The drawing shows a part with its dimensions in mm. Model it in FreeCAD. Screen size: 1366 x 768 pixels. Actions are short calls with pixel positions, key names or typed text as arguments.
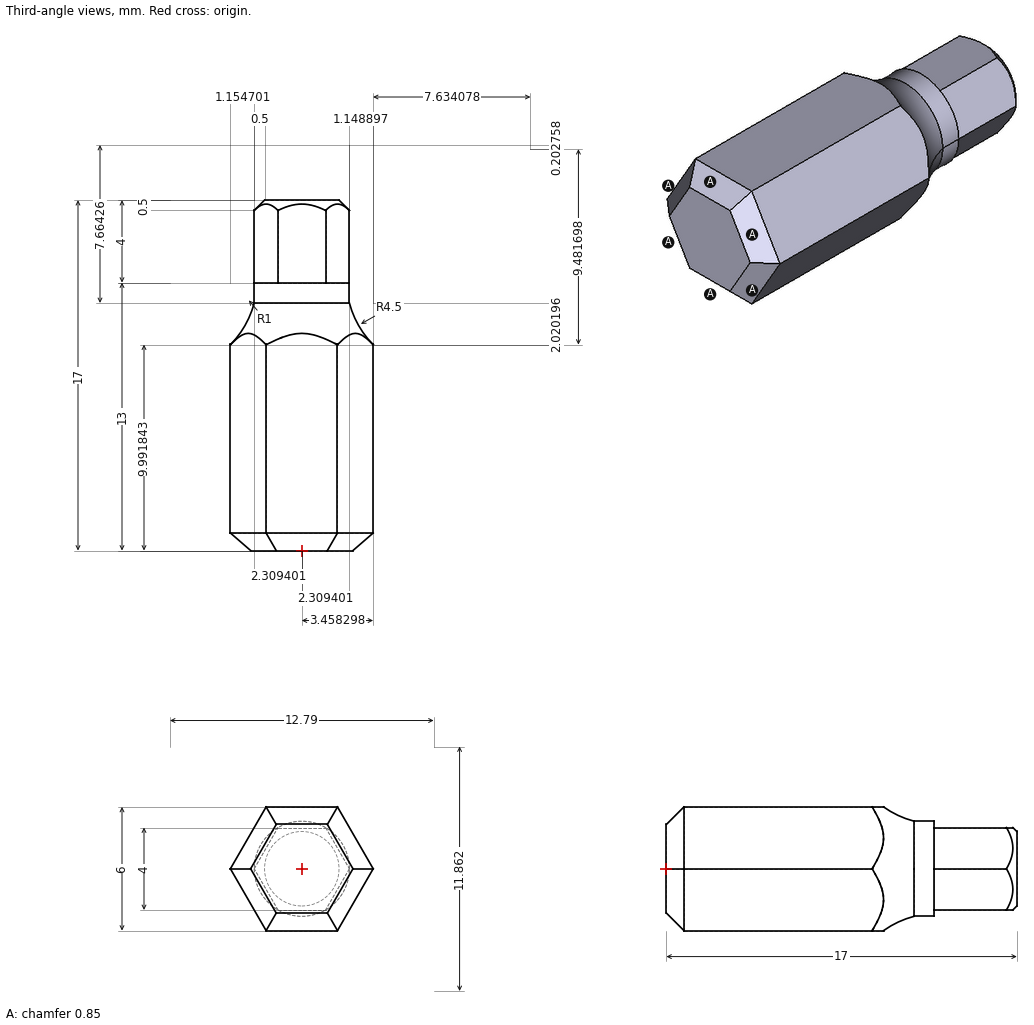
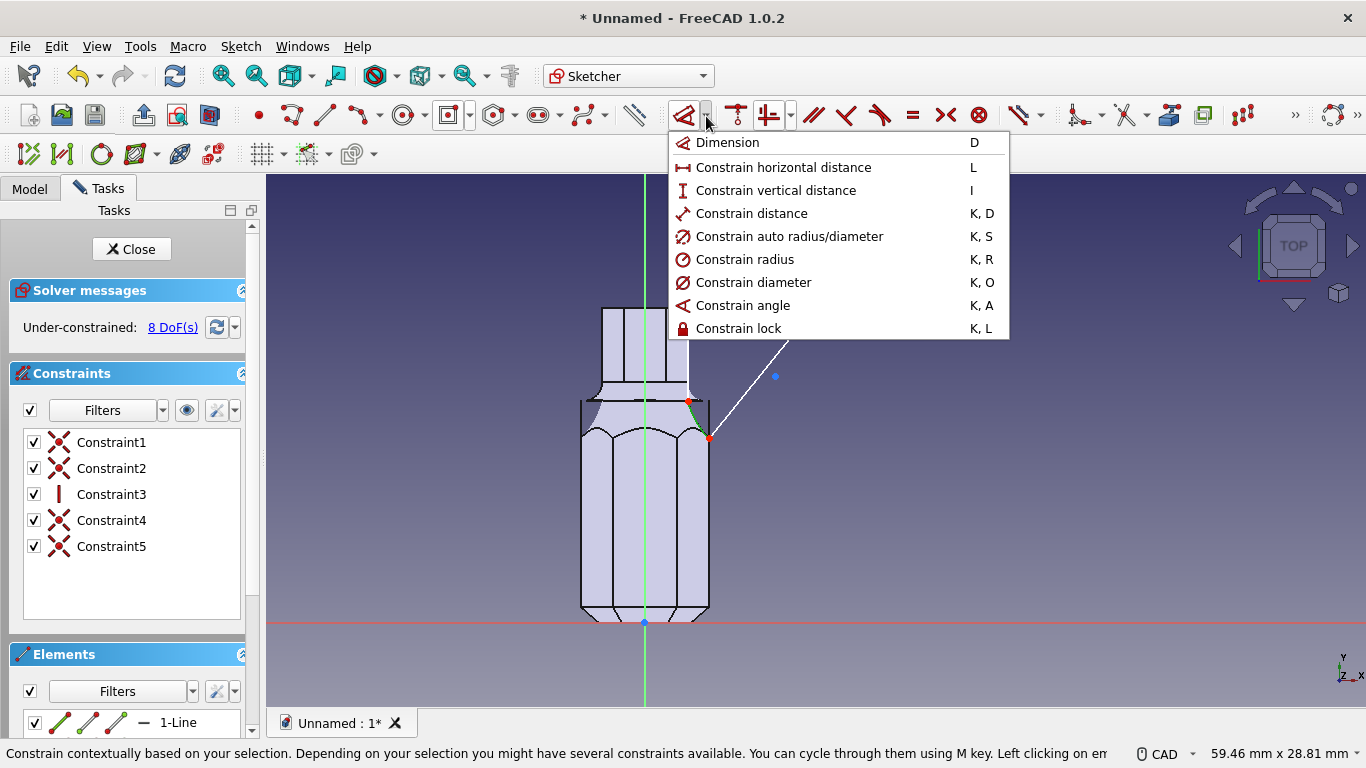
click(839, 260)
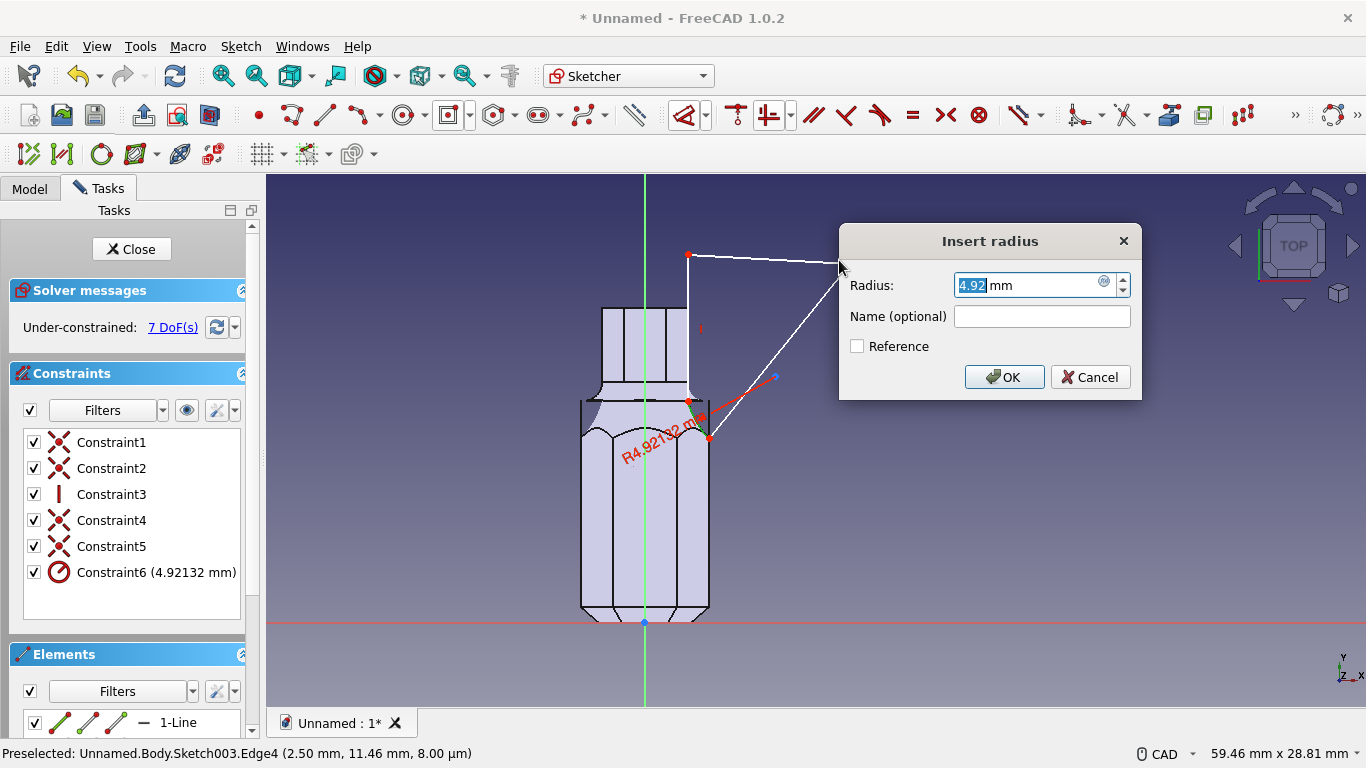
text(4.5)
key(Return)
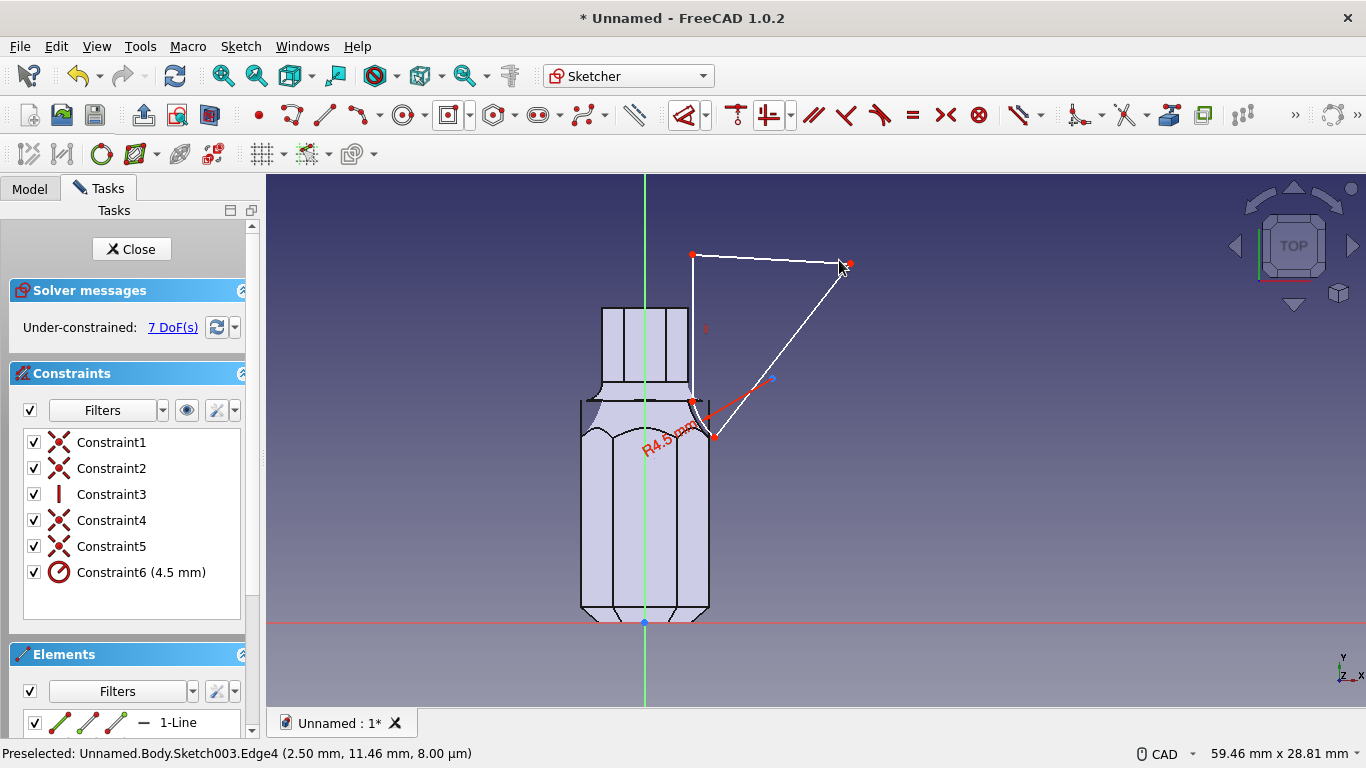
click(693, 299)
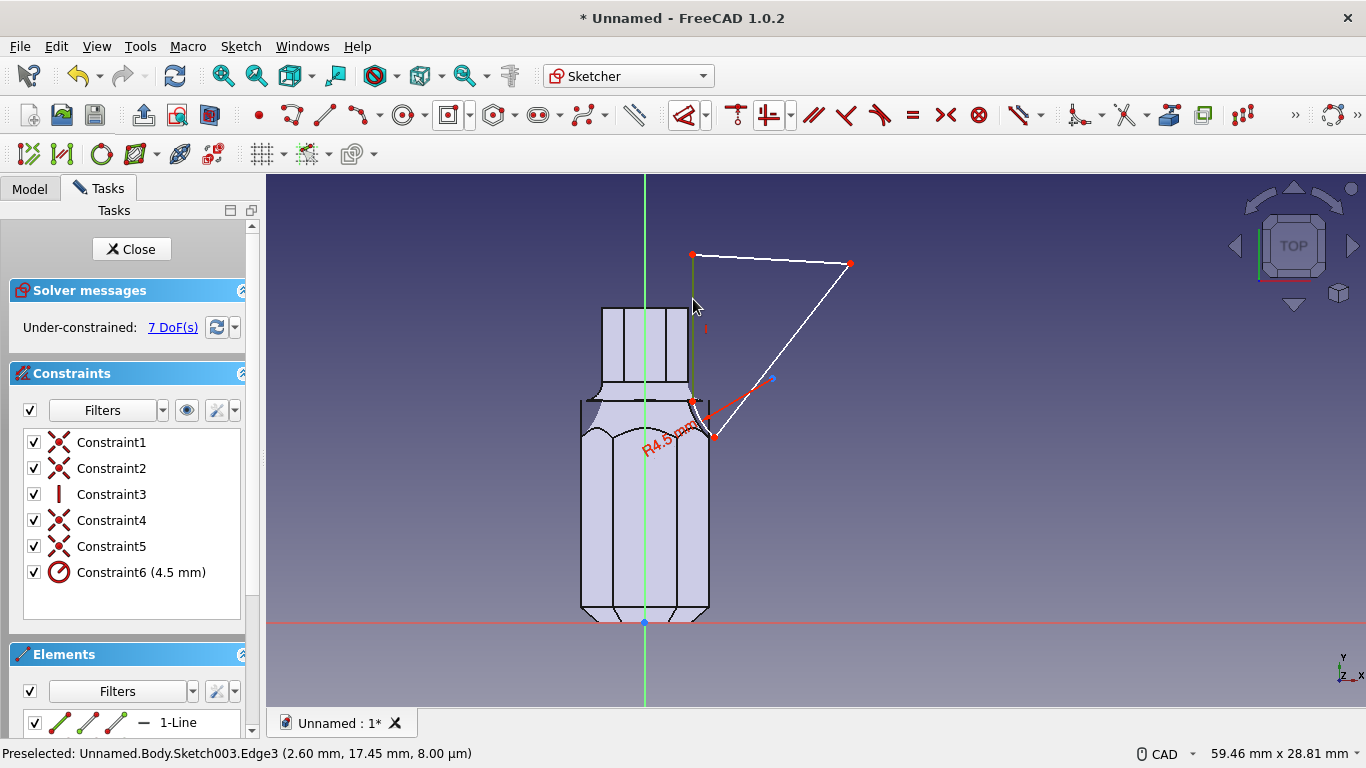
click(706, 116)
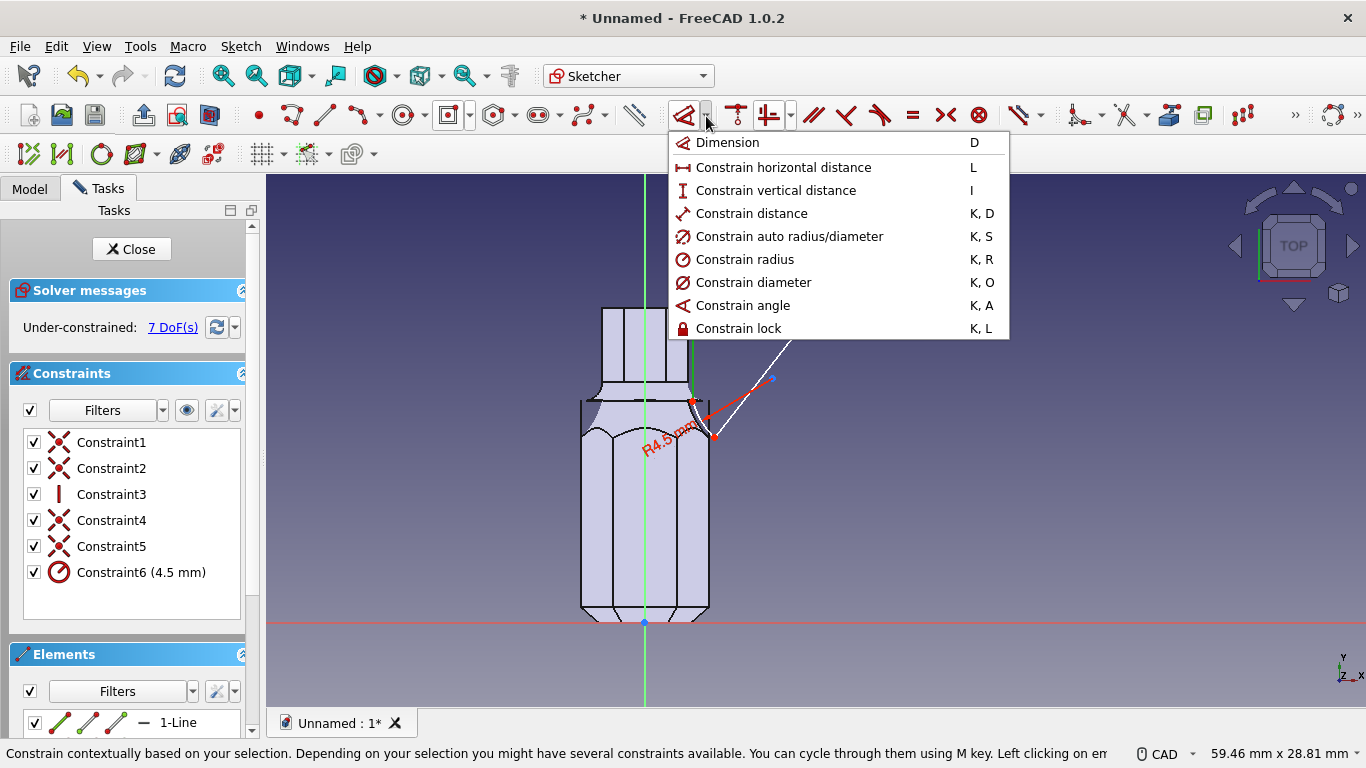
click(839, 190)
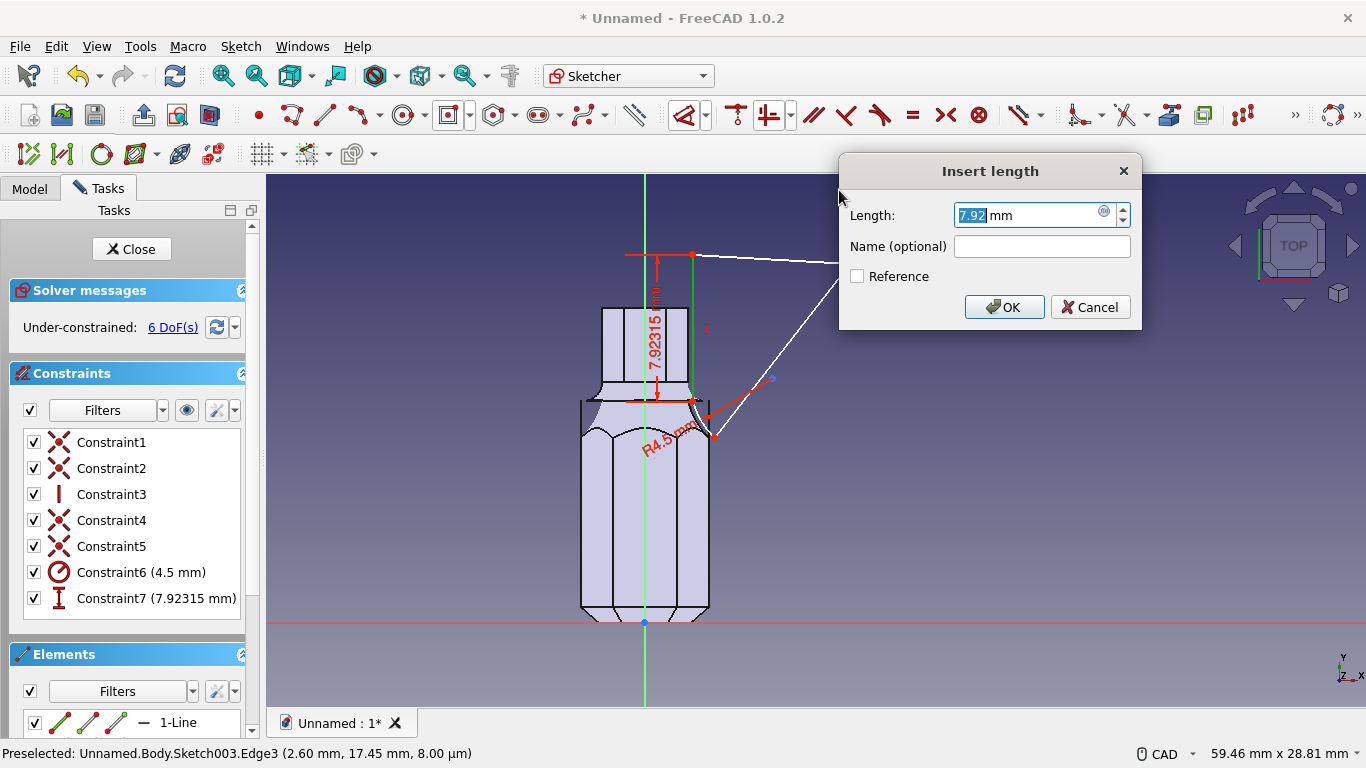
text(7.66426)
key(Return)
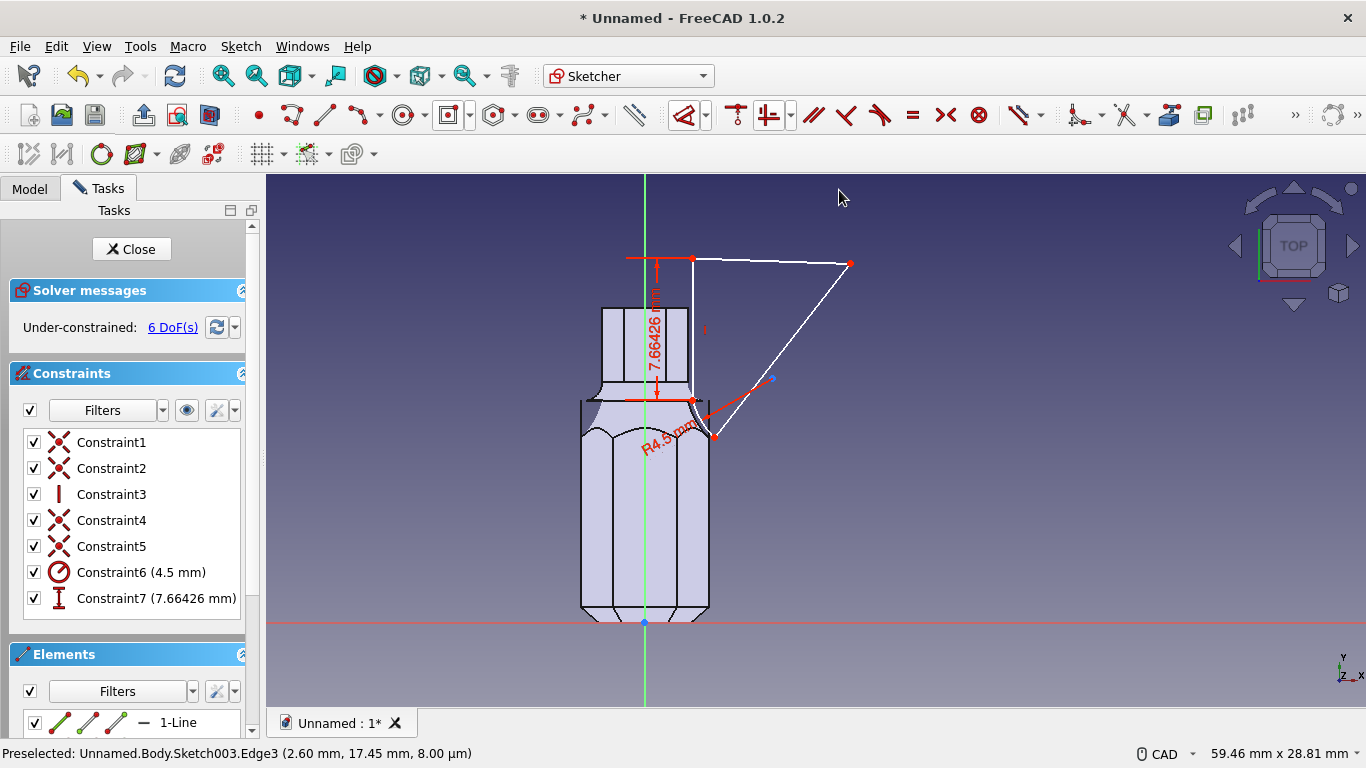
click(715, 438)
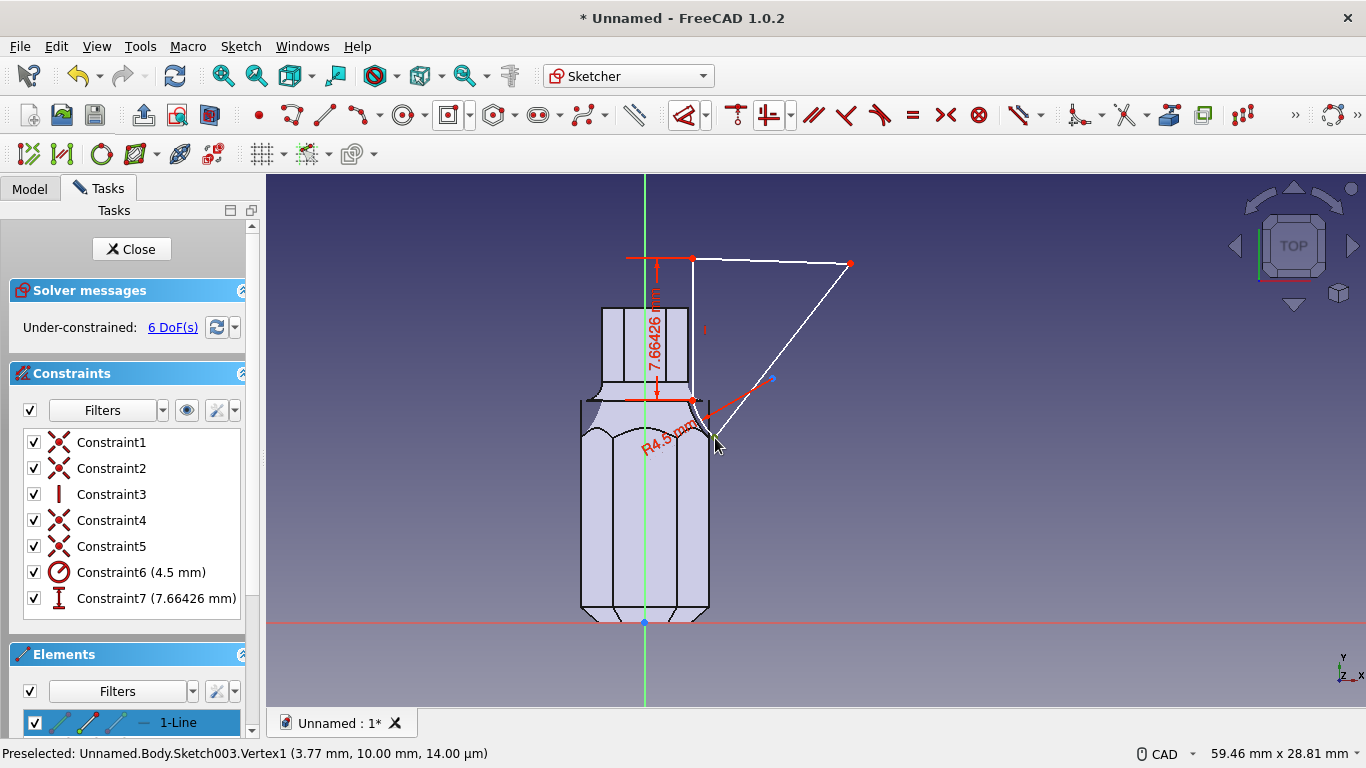
click(706, 116)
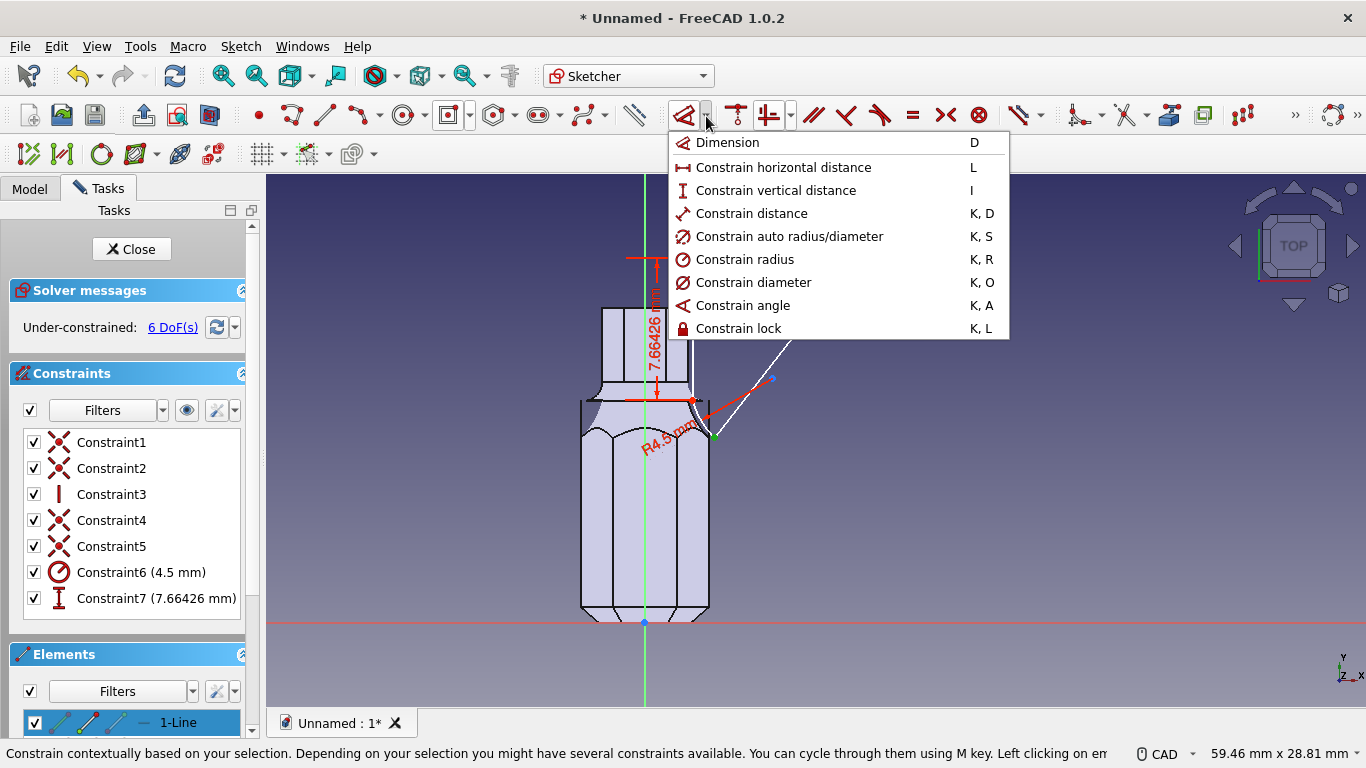
click(839, 168)